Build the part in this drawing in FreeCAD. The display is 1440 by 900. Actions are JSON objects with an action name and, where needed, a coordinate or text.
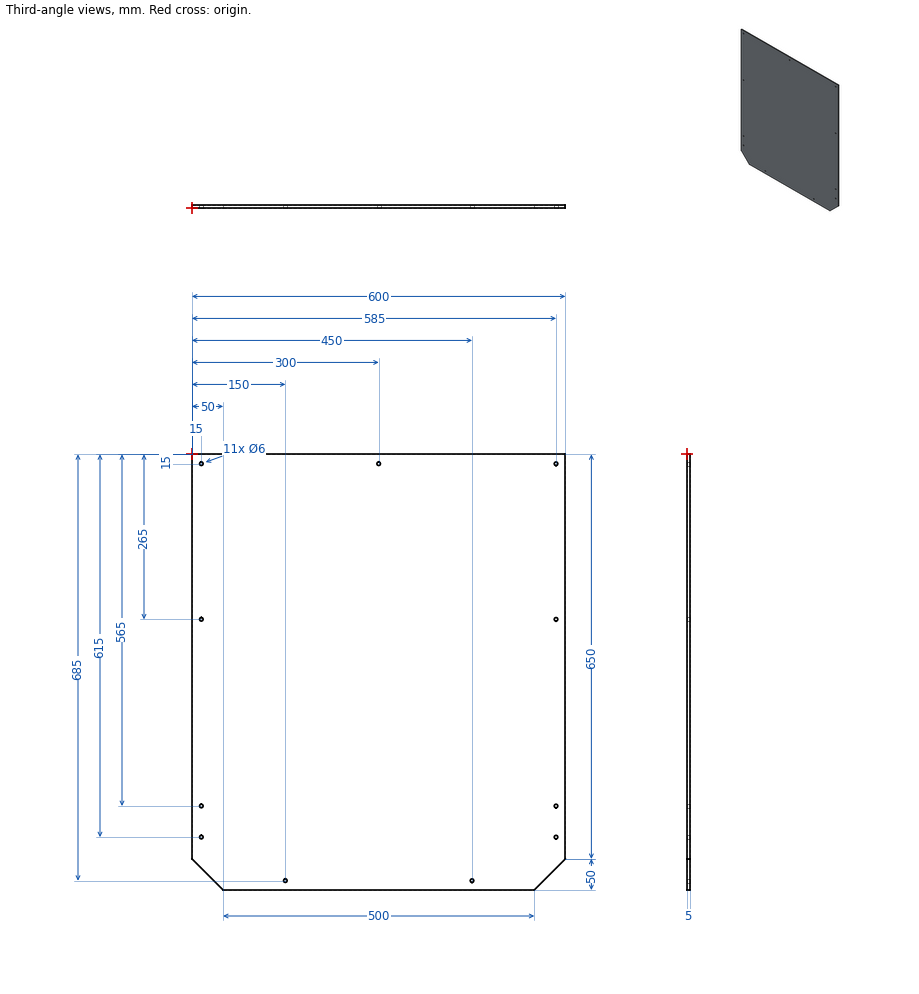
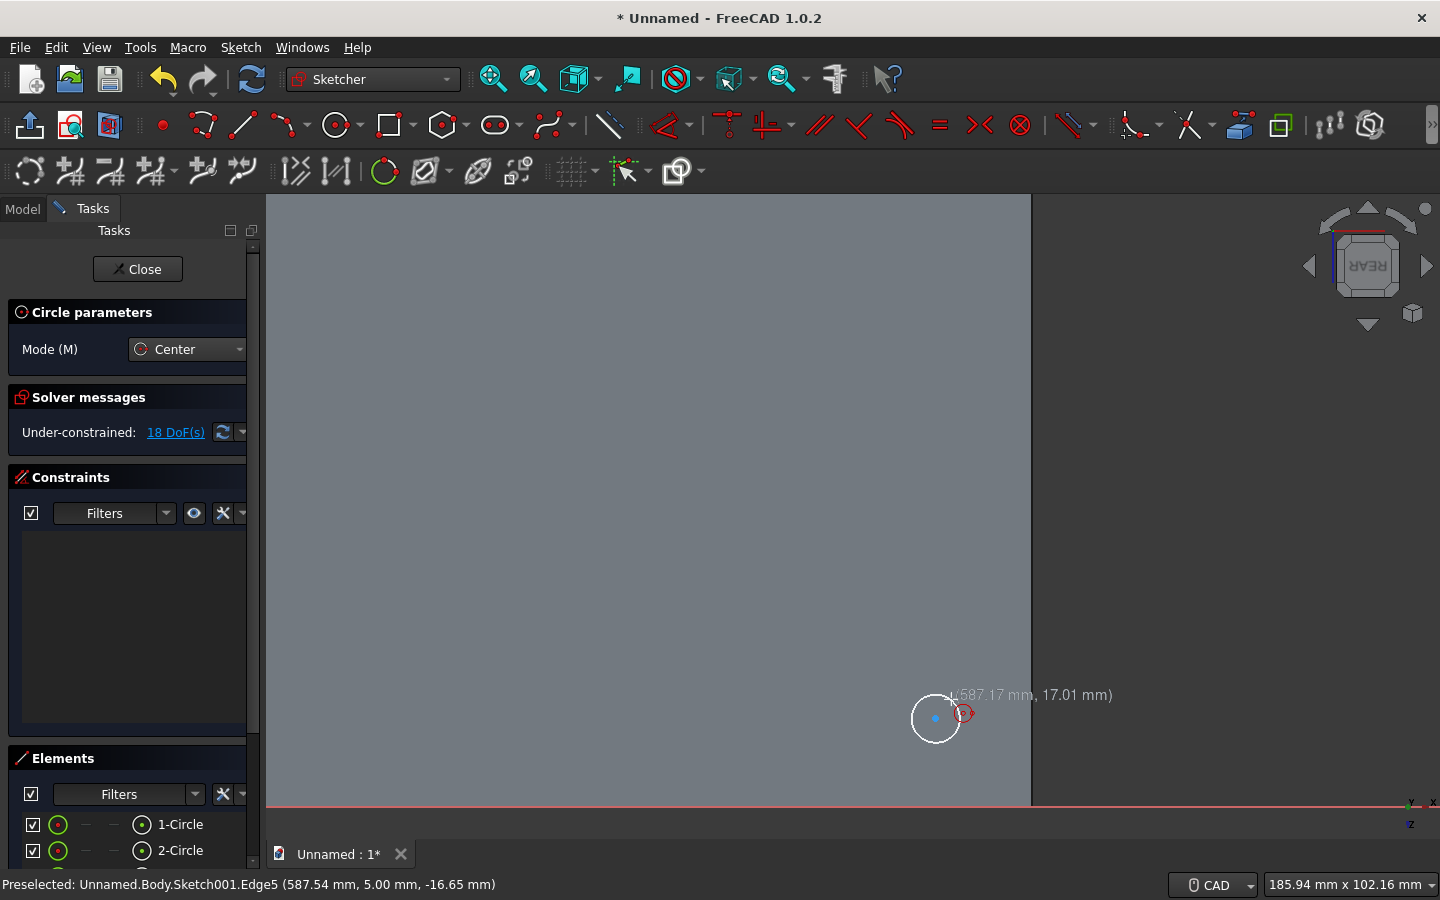
{"action": "scroll", "coordinate": [953, 704], "scroll_direction": "down", "scroll_amount": 12}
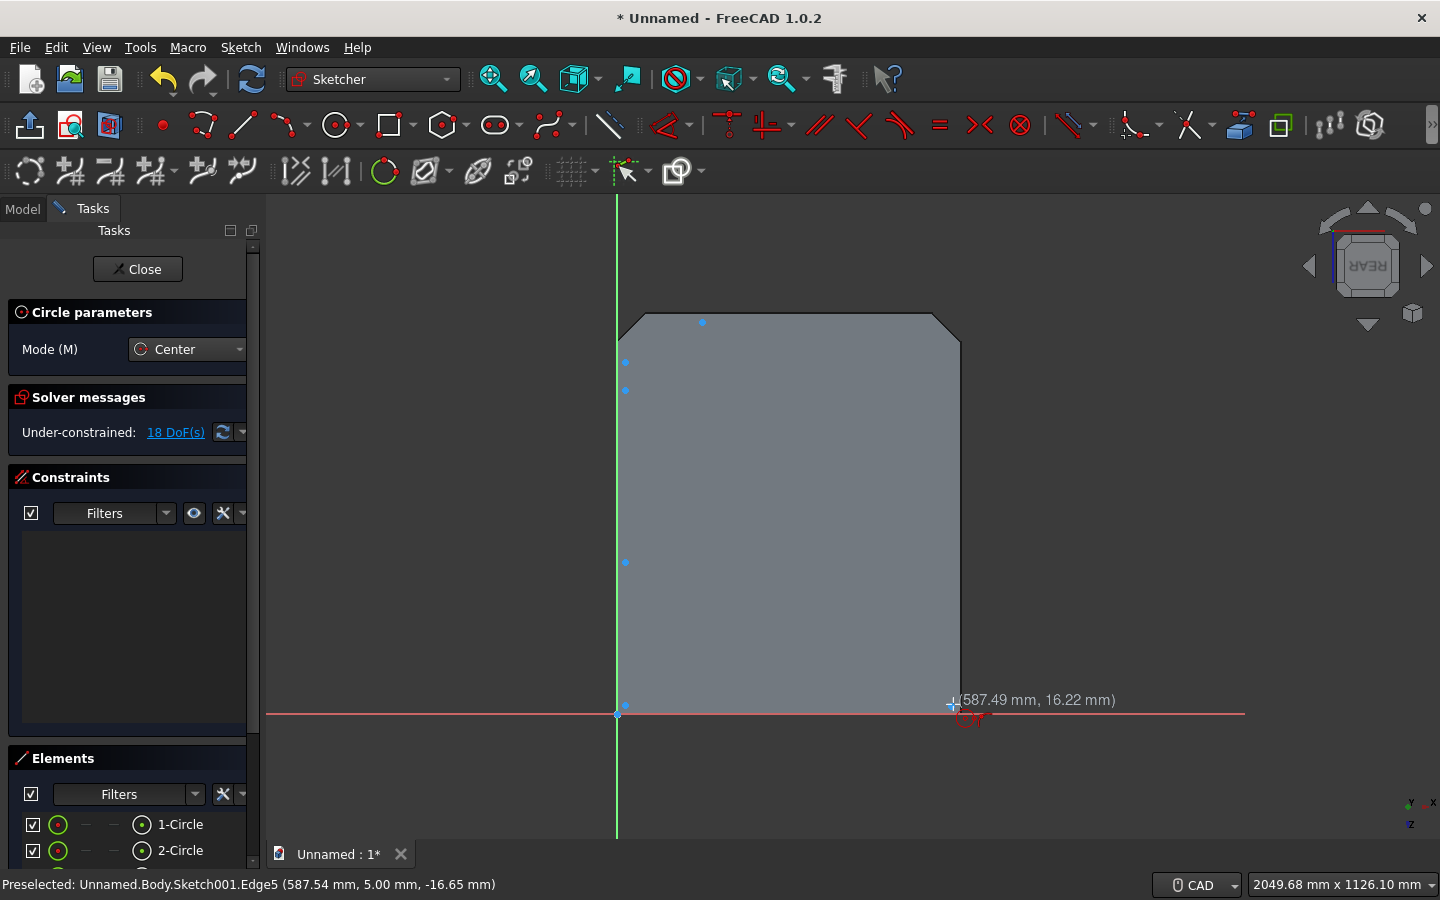
{"action": "scroll", "coordinate": [952, 562], "scroll_direction": "up", "scroll_amount": 13}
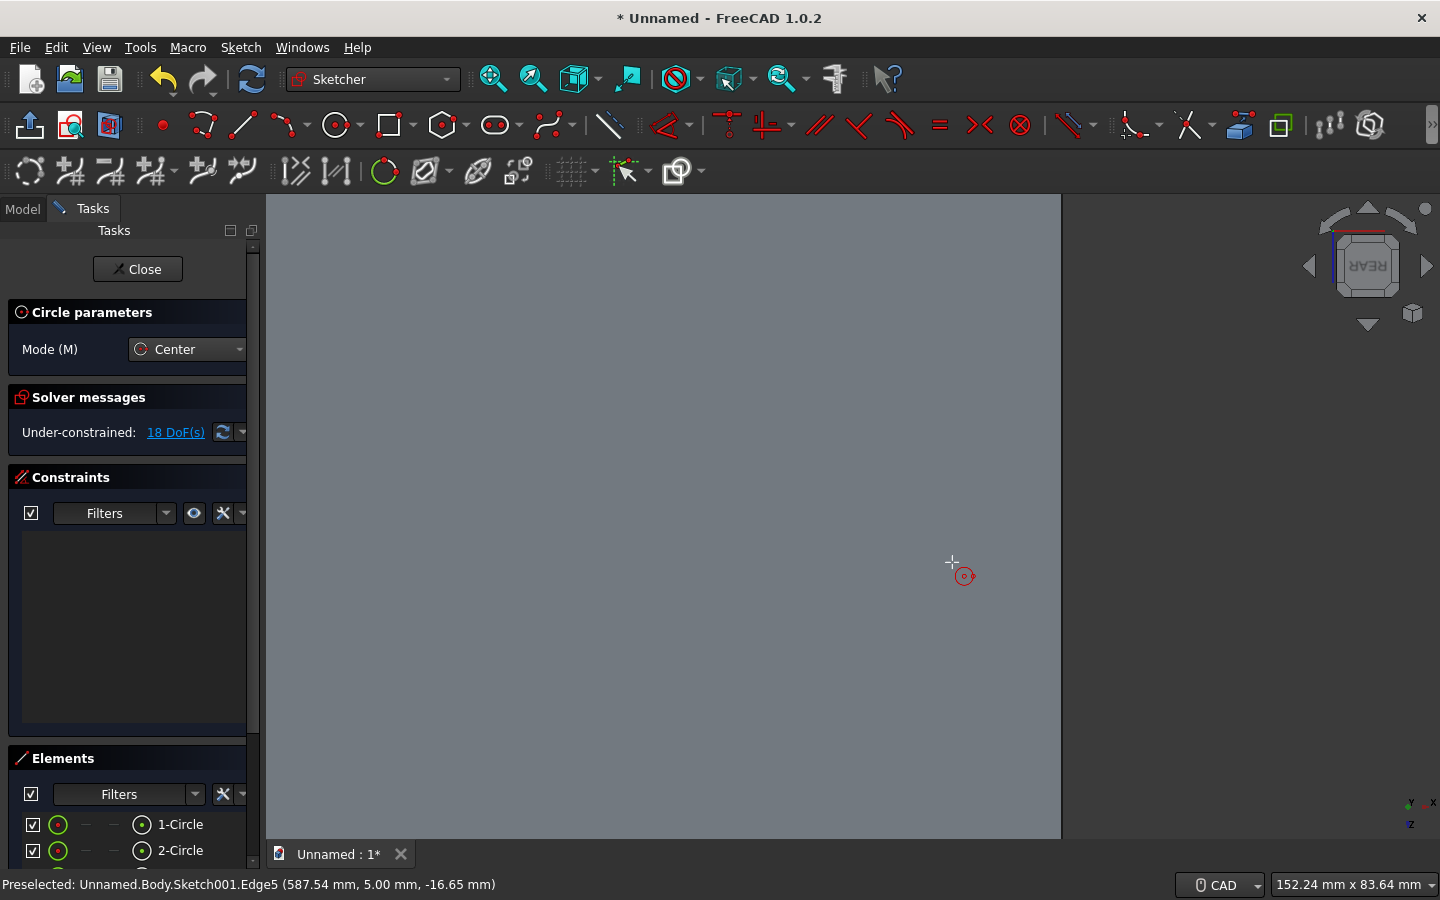
{"action": "scroll", "coordinate": [952, 562], "scroll_direction": "down", "scroll_amount": 13}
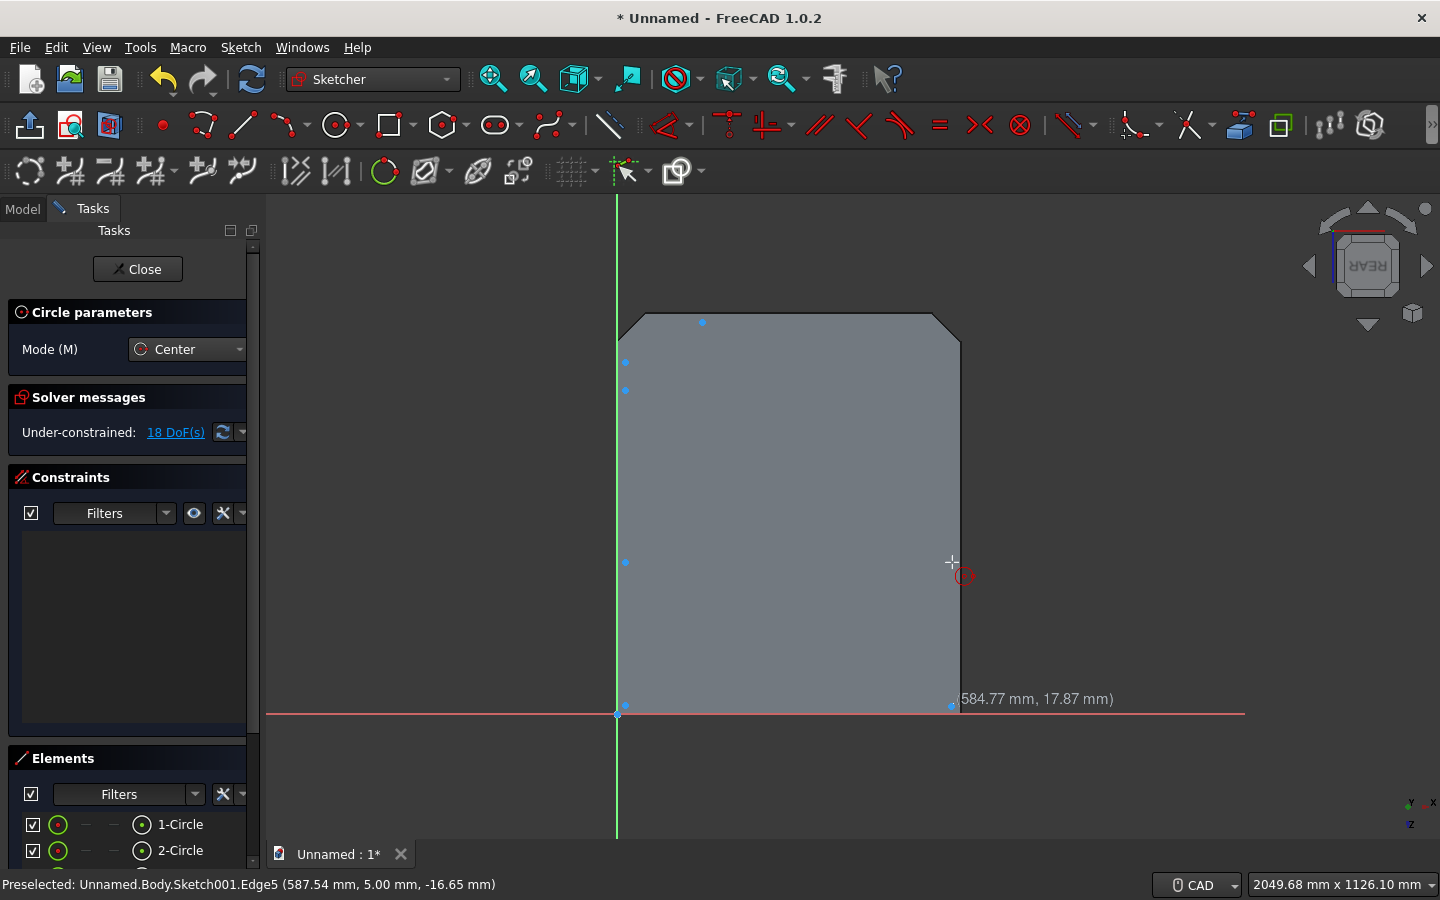
{"action": "left_click", "coordinate": [952, 562]}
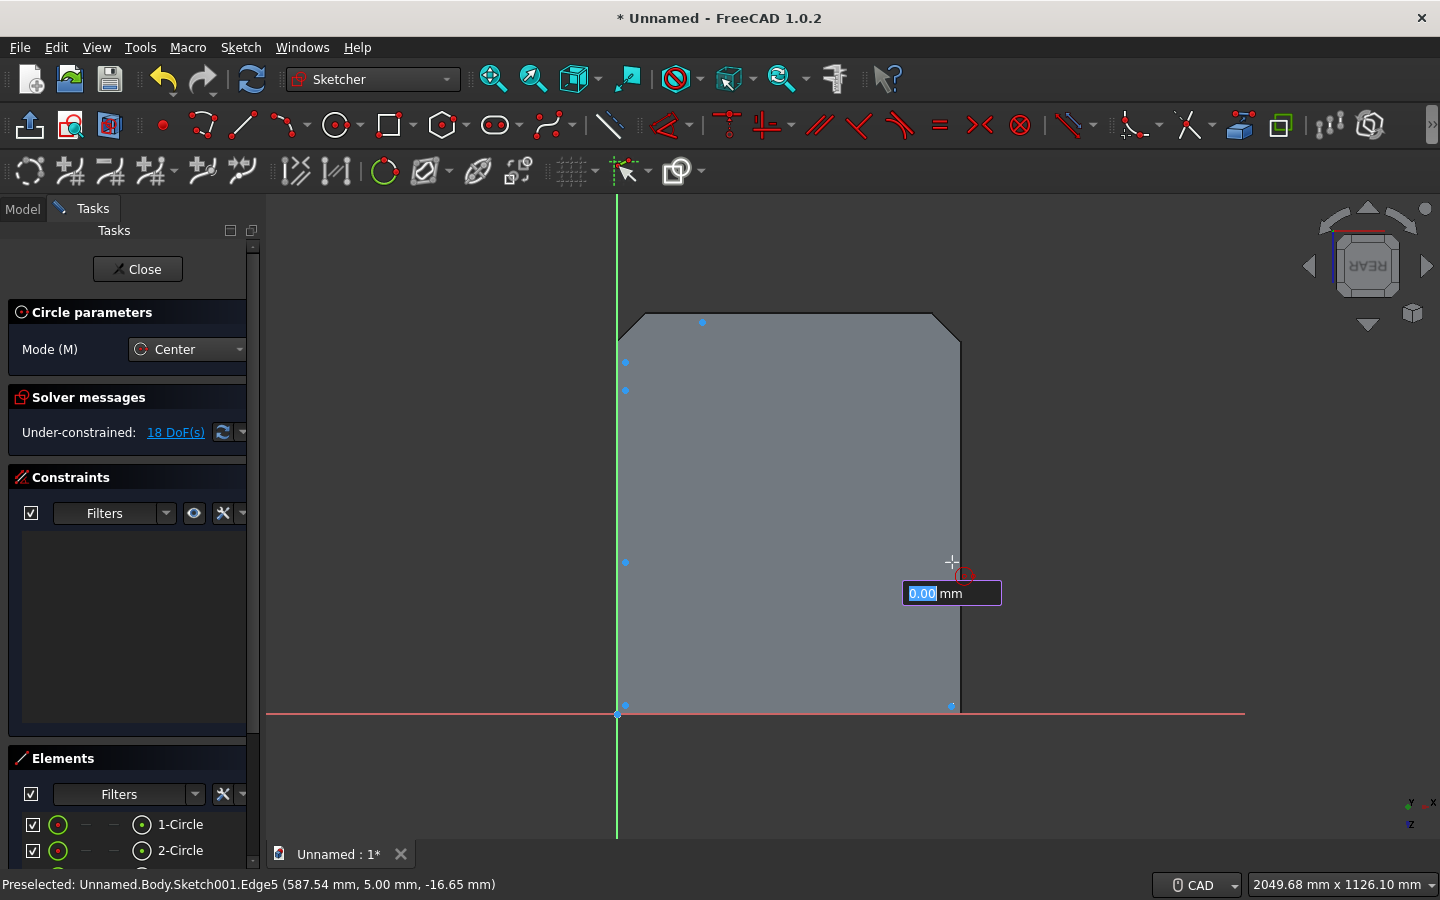
{"action": "scroll", "coordinate": [953, 561], "scroll_direction": "up", "scroll_amount": 12}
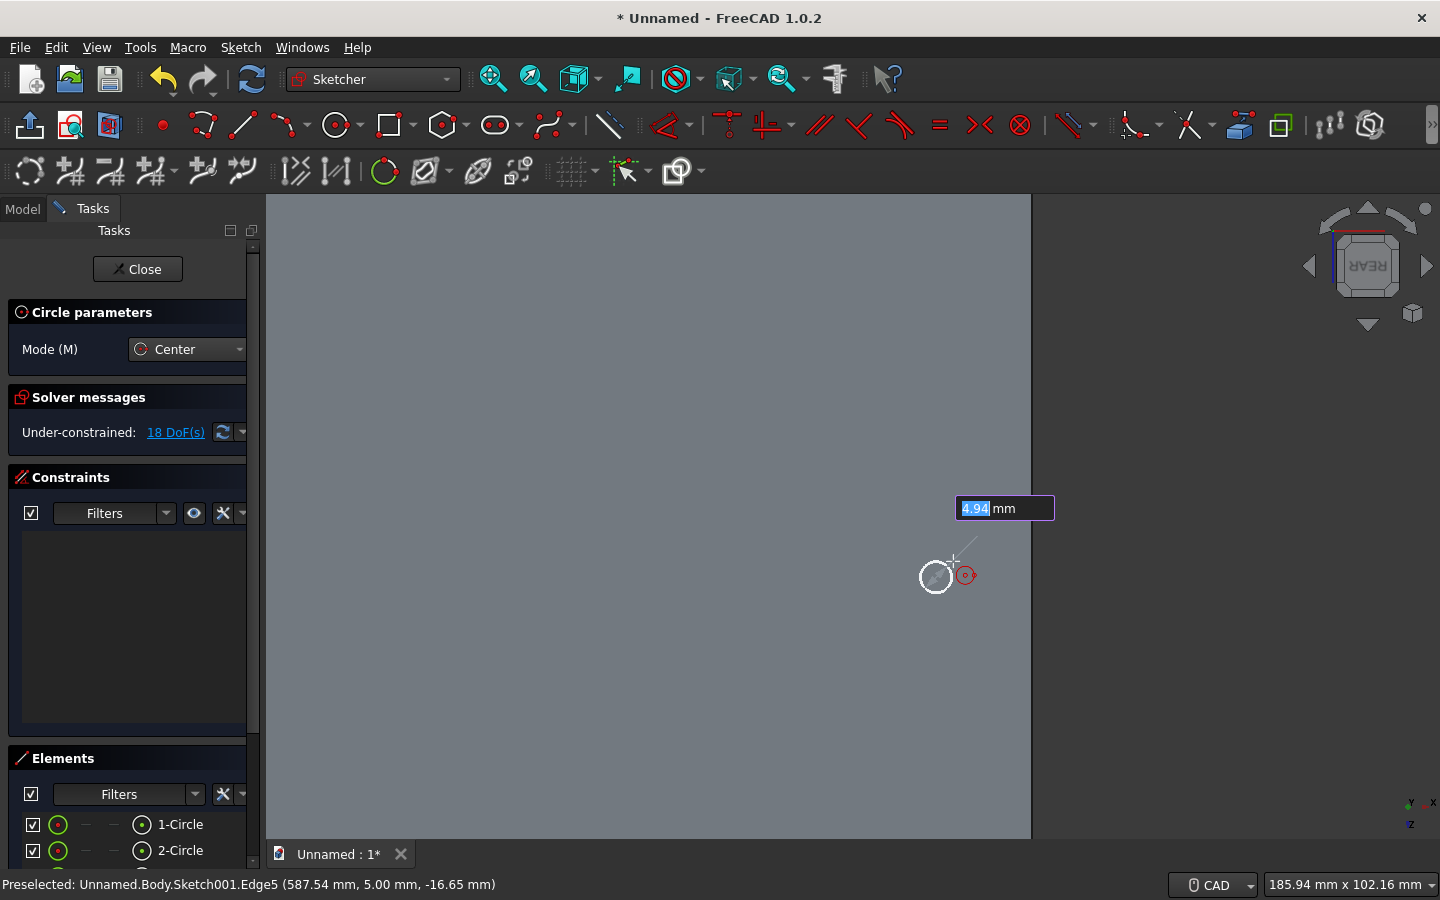
{"action": "left_click", "coordinate": [951, 556]}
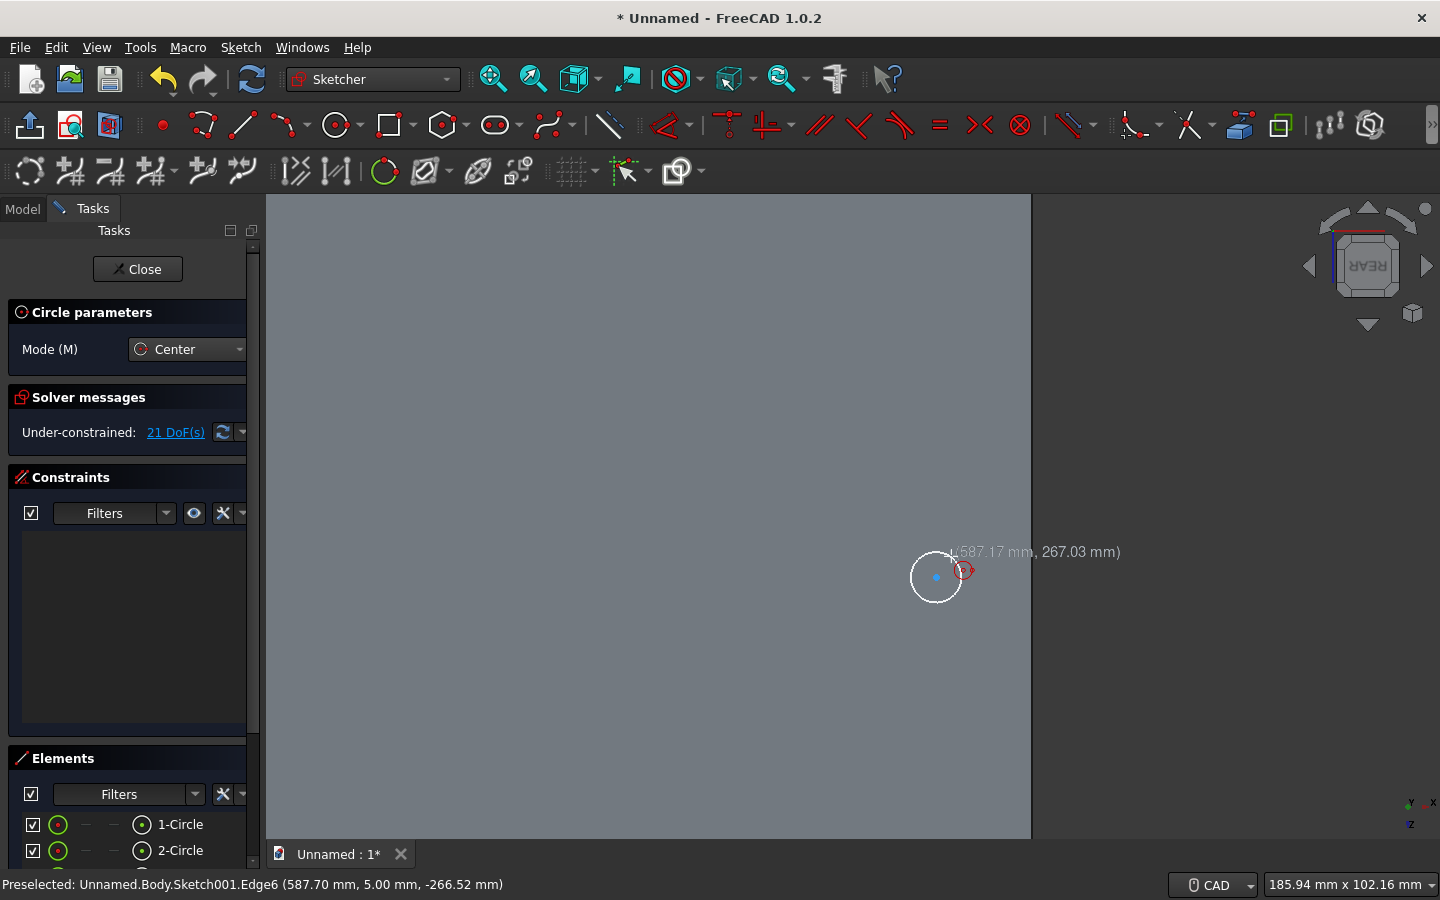
{"action": "scroll", "coordinate": [953, 561], "scroll_direction": "down", "scroll_amount": 12}